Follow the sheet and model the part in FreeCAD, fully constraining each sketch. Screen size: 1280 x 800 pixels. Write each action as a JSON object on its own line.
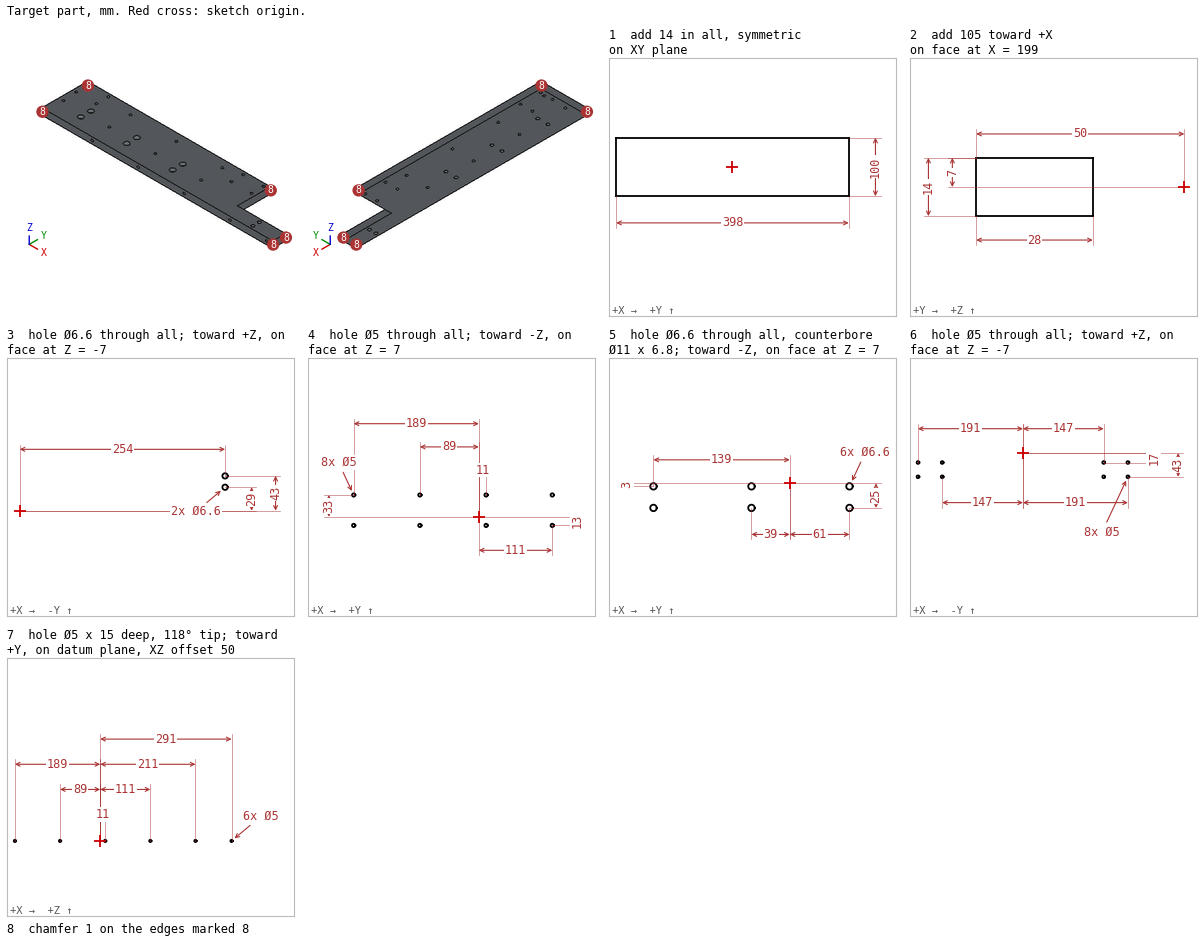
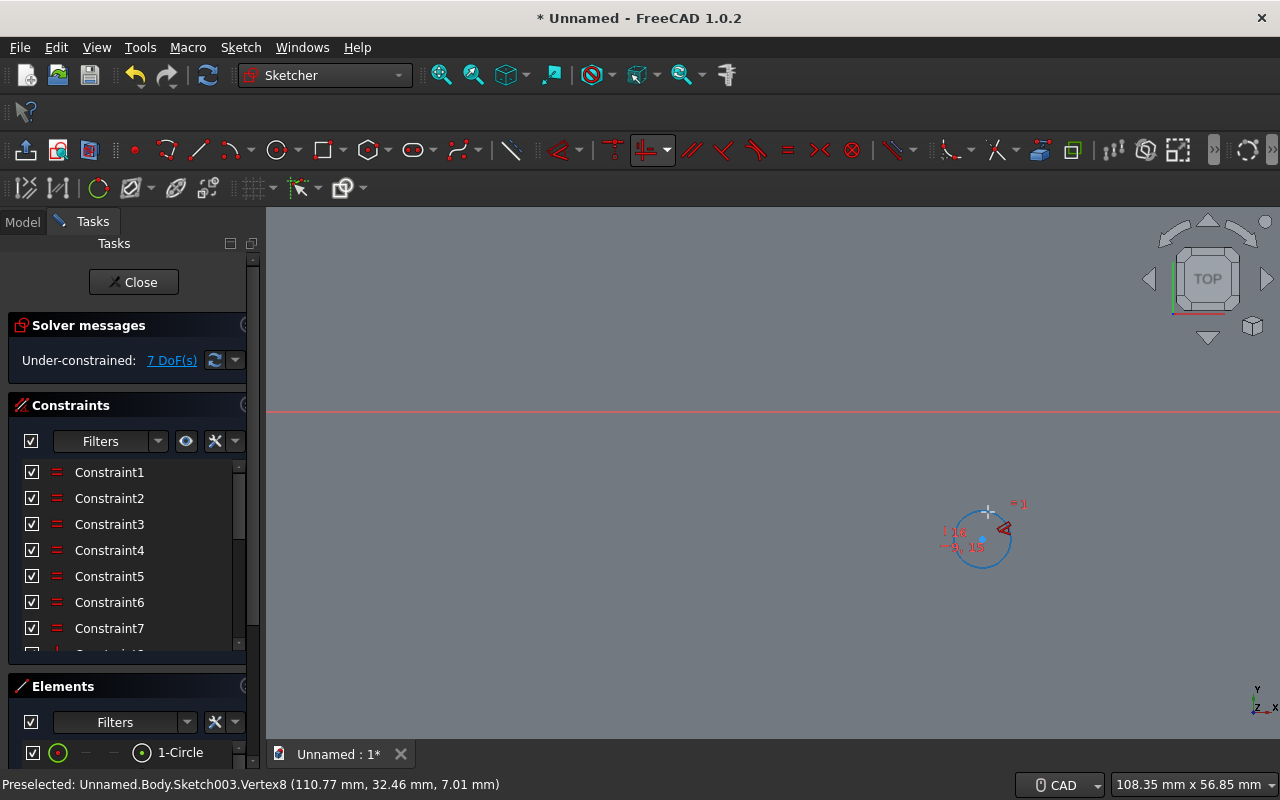
{"action": "left_click", "coordinate": [983, 511]}
{"action": "left_click", "coordinate": [984, 479]}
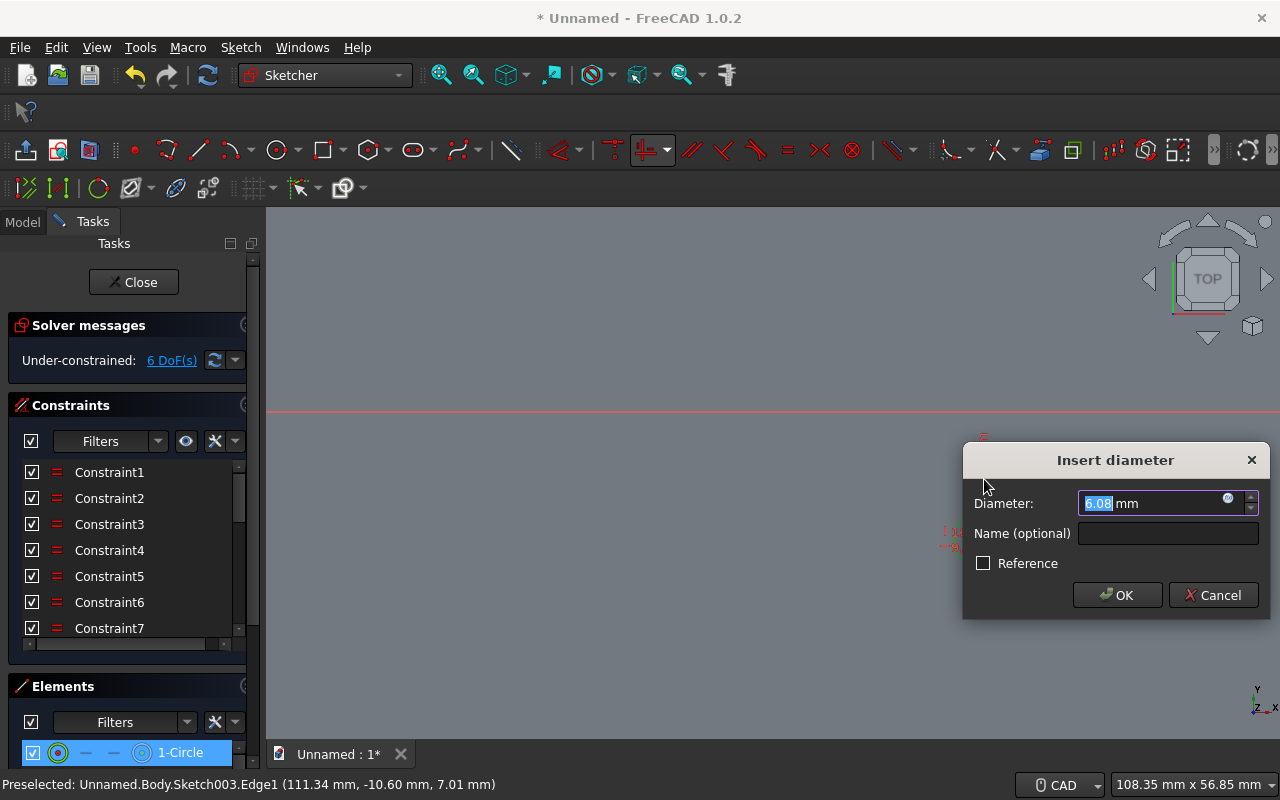
{"action": "type", "text": "5"}
{"action": "key", "text": "Return"}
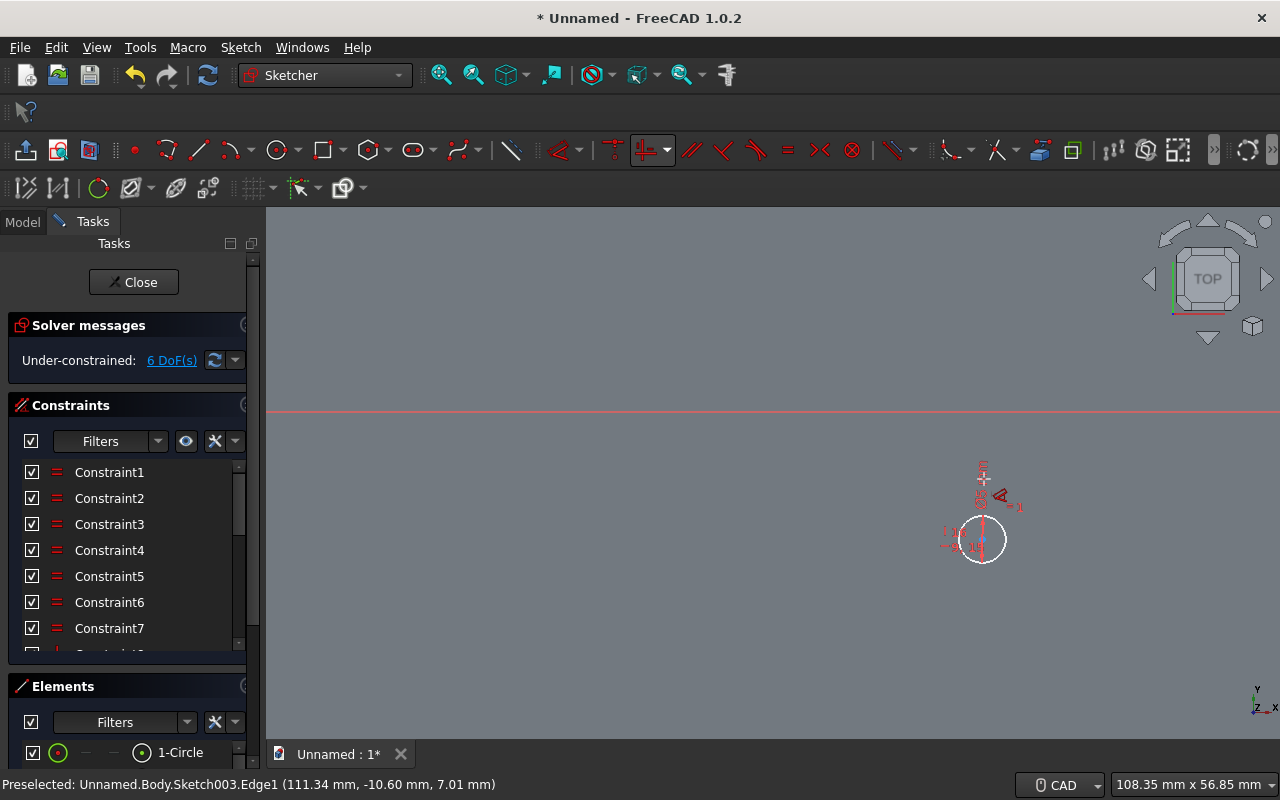
{"action": "scroll", "coordinate": [989, 512], "scroll_direction": "down", "scroll_amount": 8}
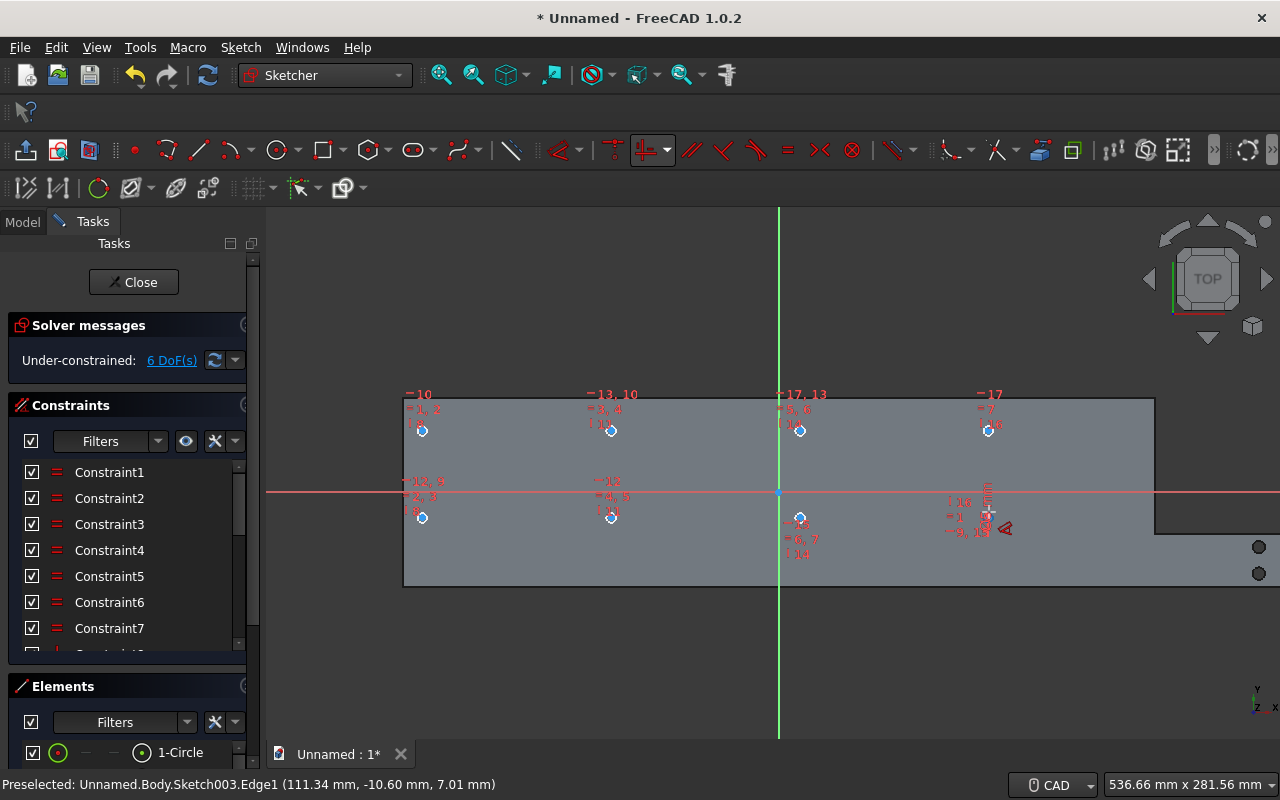
{"action": "scroll", "coordinate": [988, 518], "scroll_direction": "up", "scroll_amount": 3}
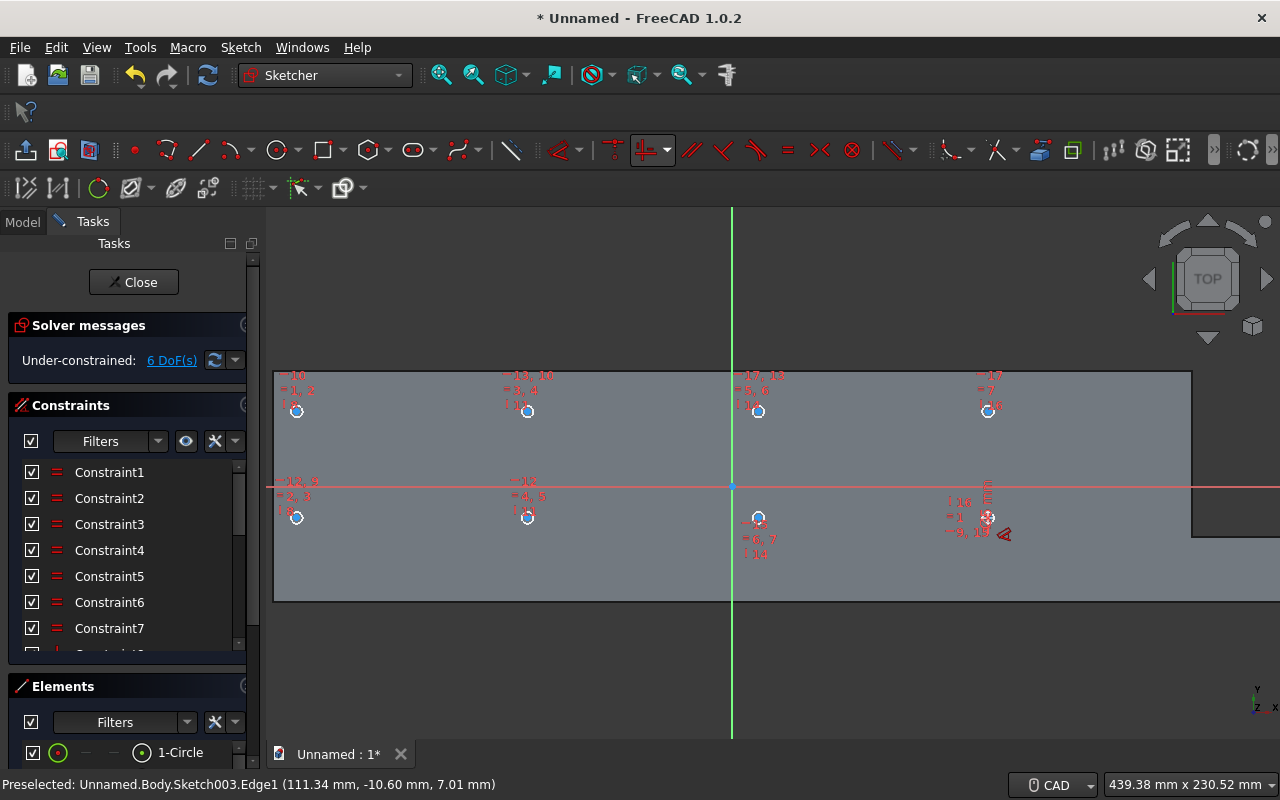
{"action": "left_click", "coordinate": [988, 518]}
{"action": "left_click", "coordinate": [572, 494]}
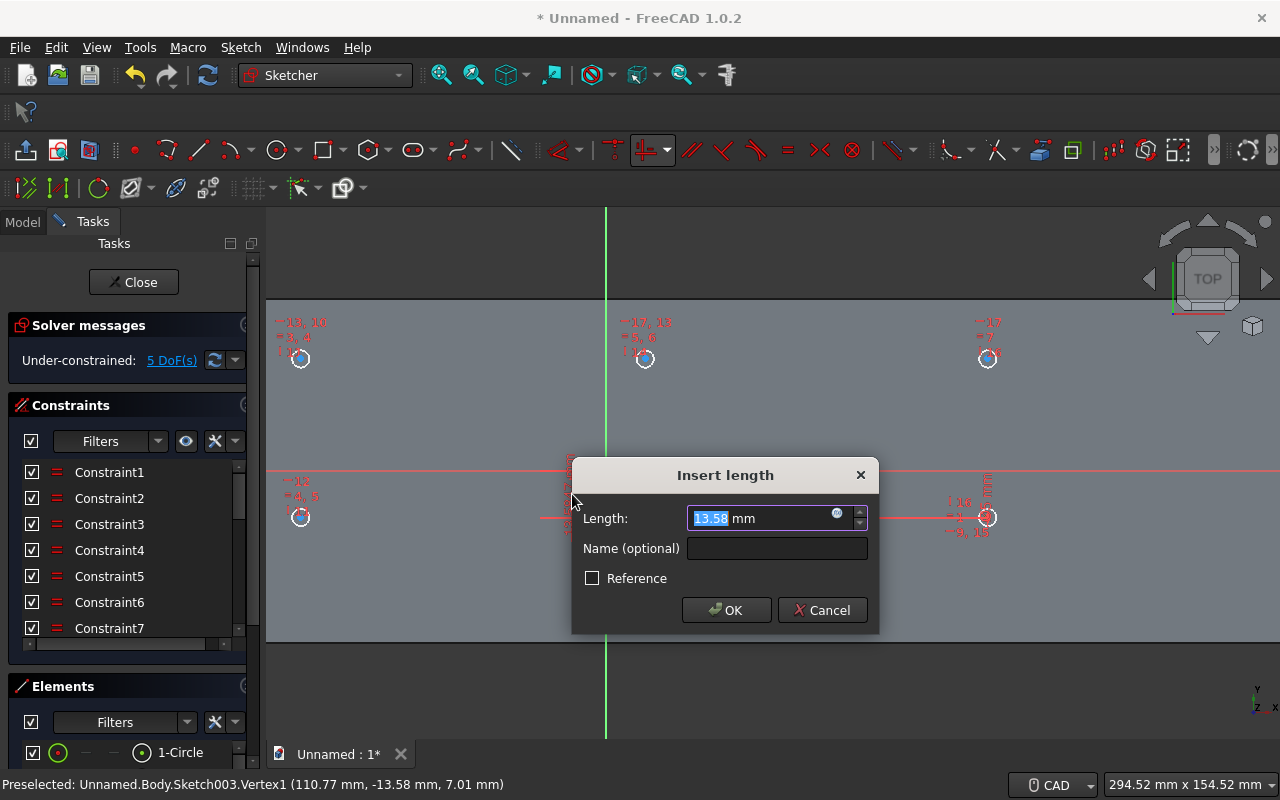
{"action": "type", "text": "13"}
{"action": "key", "text": "Return"}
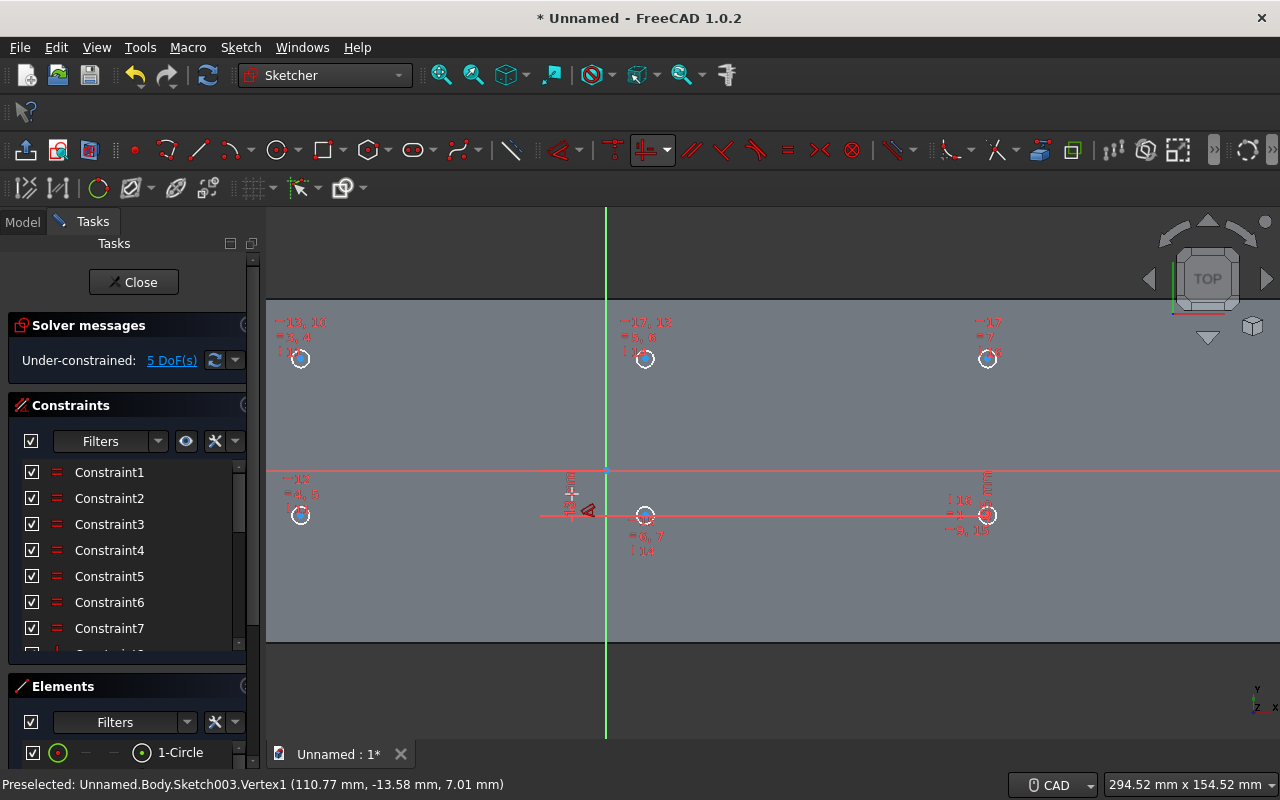
{"action": "scroll", "coordinate": [987, 518], "scroll_direction": "down", "scroll_amount": 3}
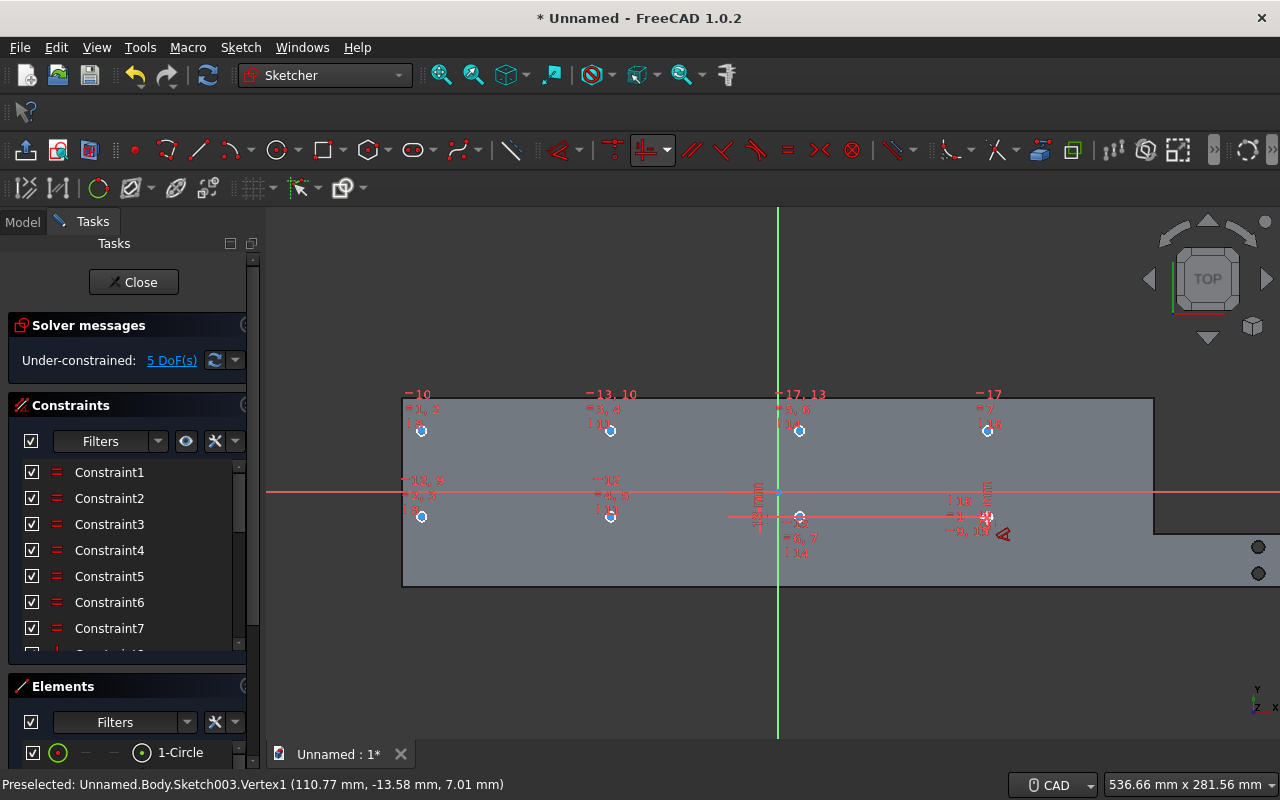
{"action": "left_click", "coordinate": [422, 431]}
{"action": "left_click", "coordinate": [388, 462]}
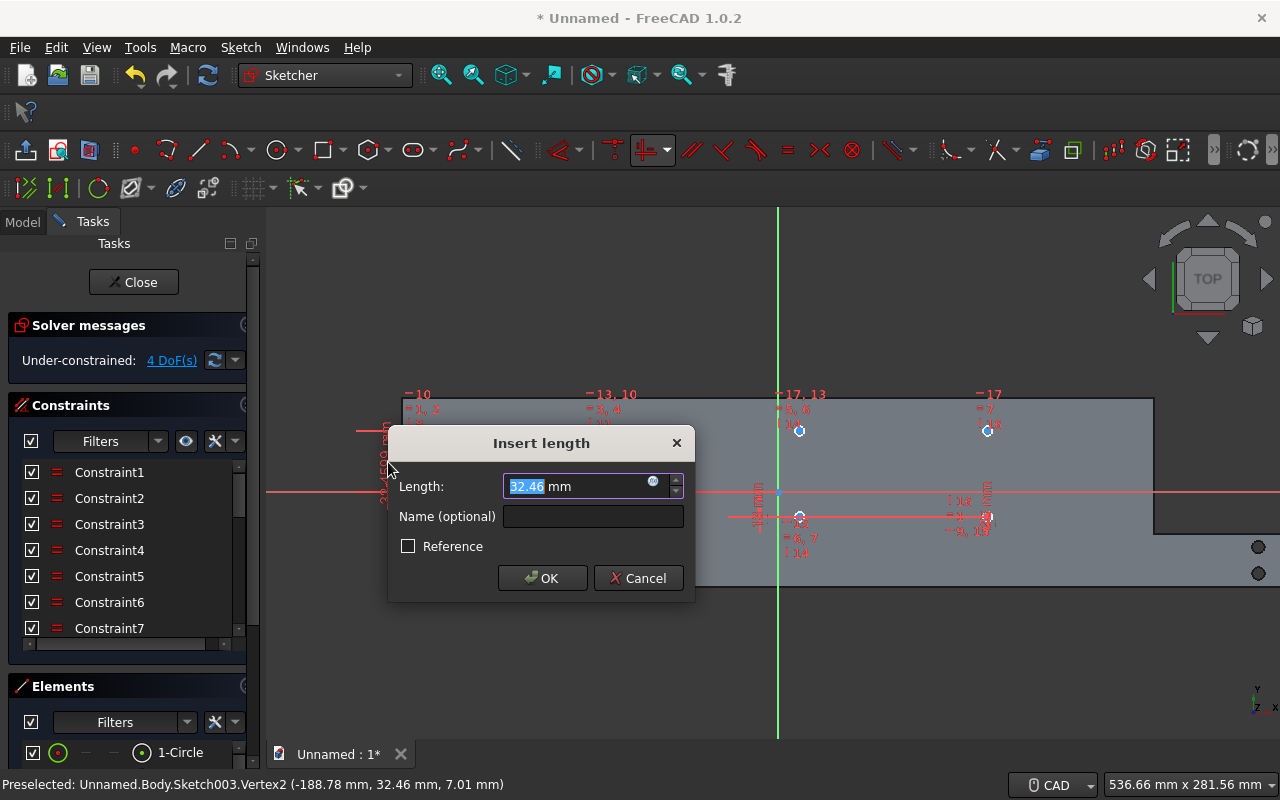
{"action": "type", "text": "33"}
{"action": "key", "text": "Return"}